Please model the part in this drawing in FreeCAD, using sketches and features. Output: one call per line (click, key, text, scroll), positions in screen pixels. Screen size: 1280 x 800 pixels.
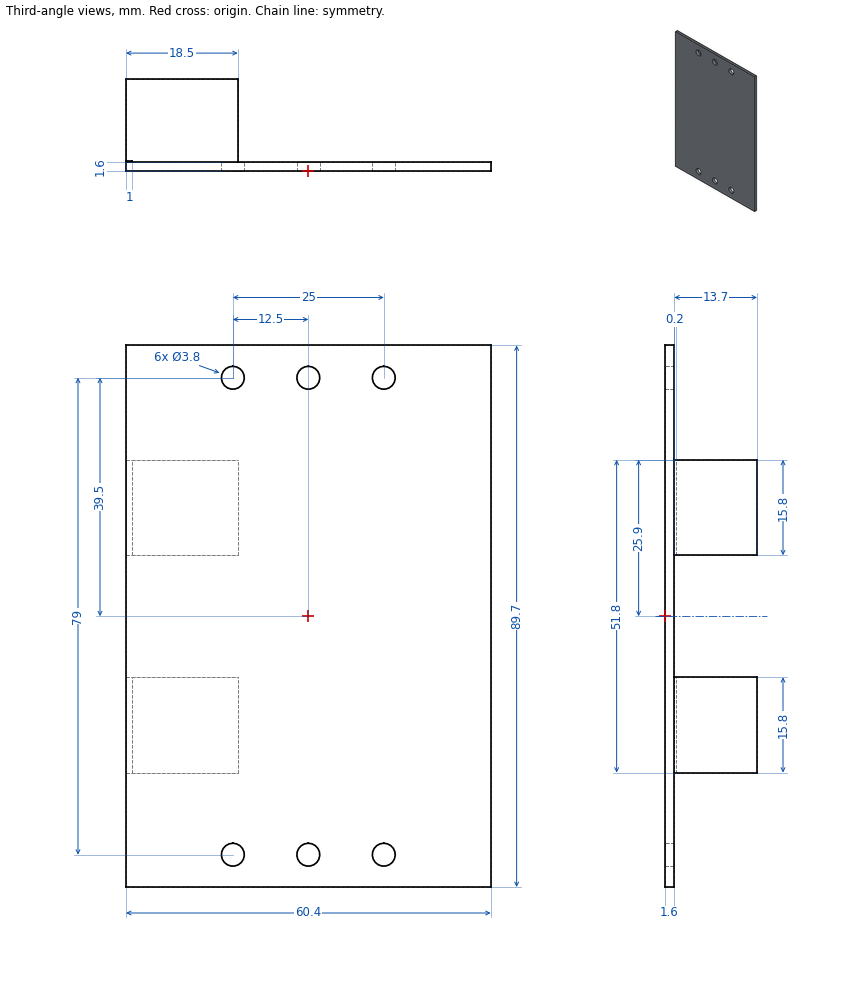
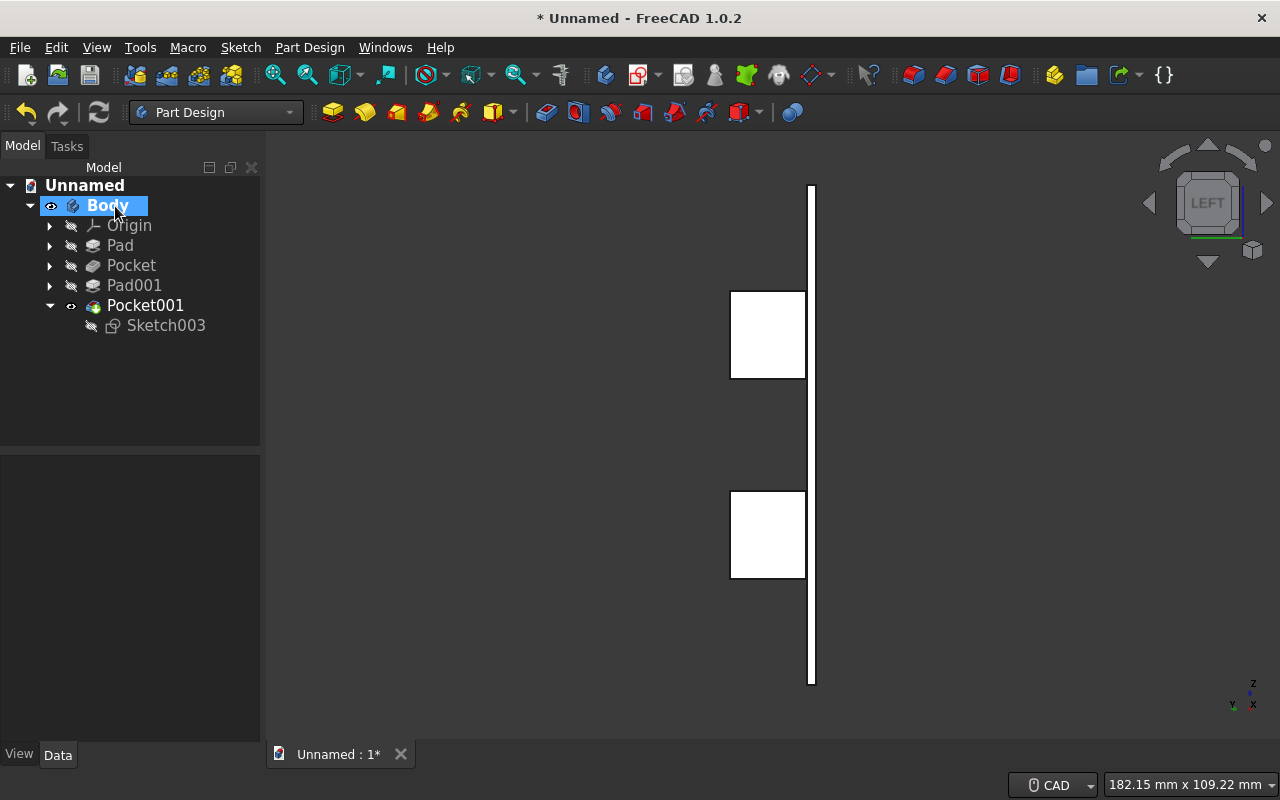
key(0)